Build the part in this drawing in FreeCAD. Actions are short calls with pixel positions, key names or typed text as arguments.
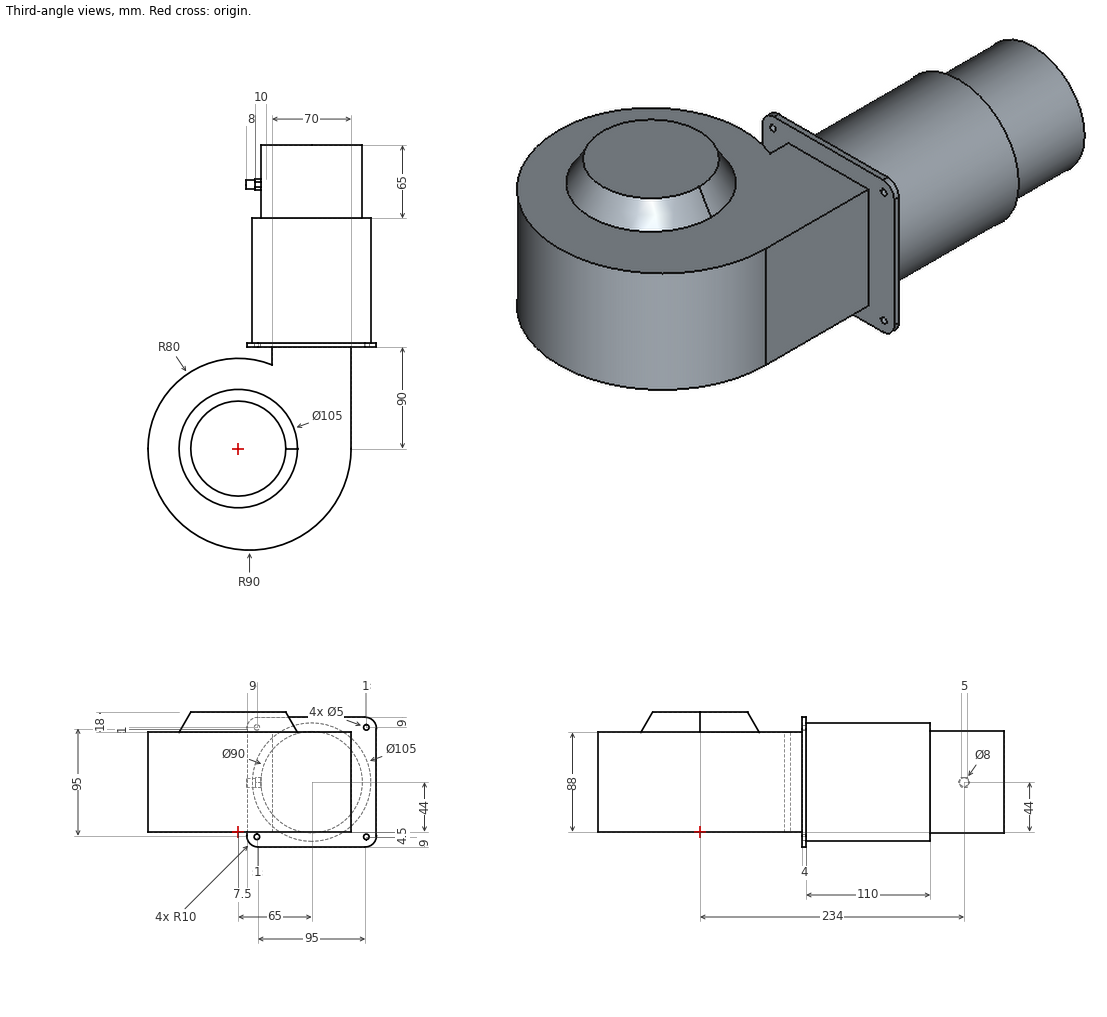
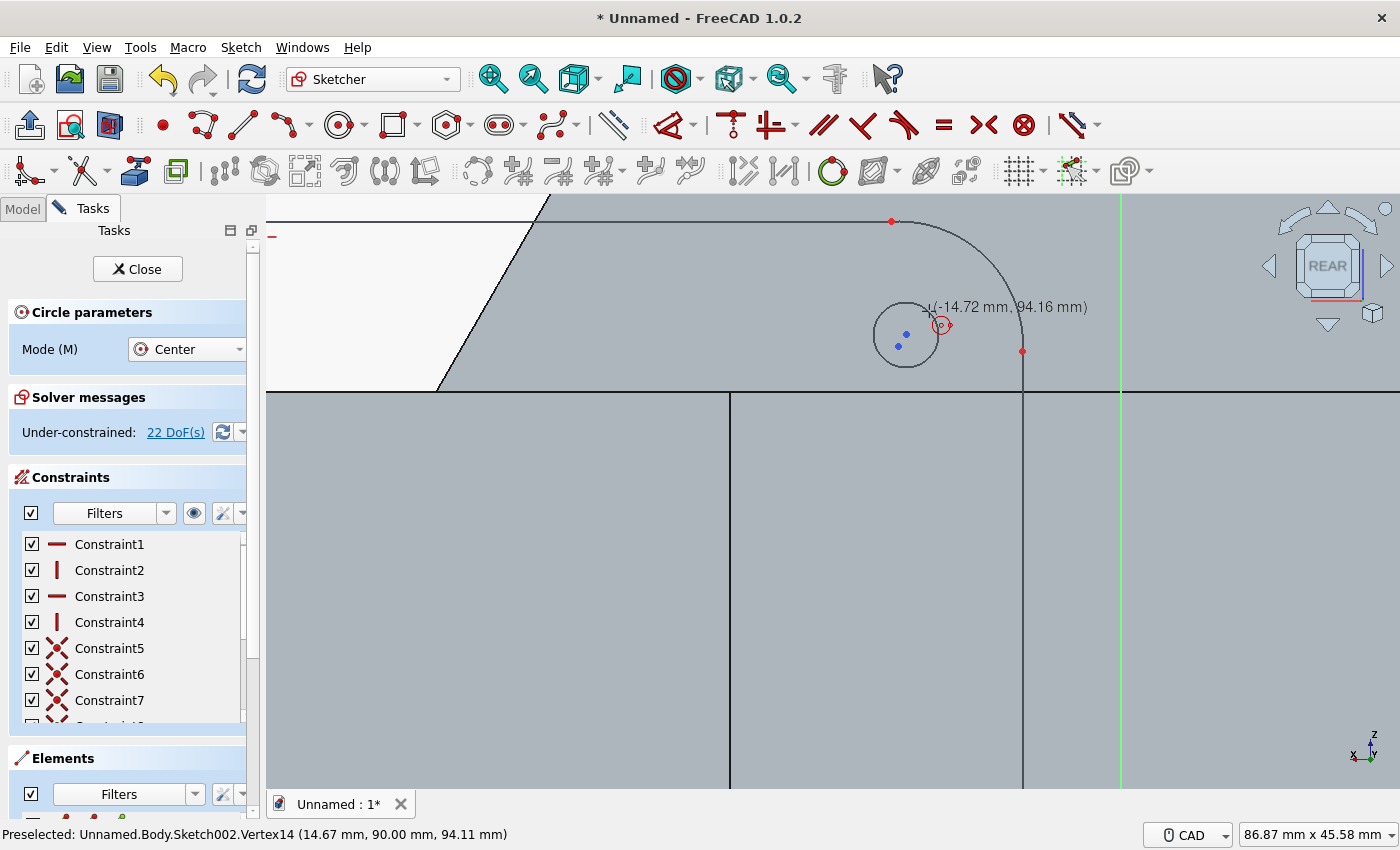
scroll(909, 336, down, 7)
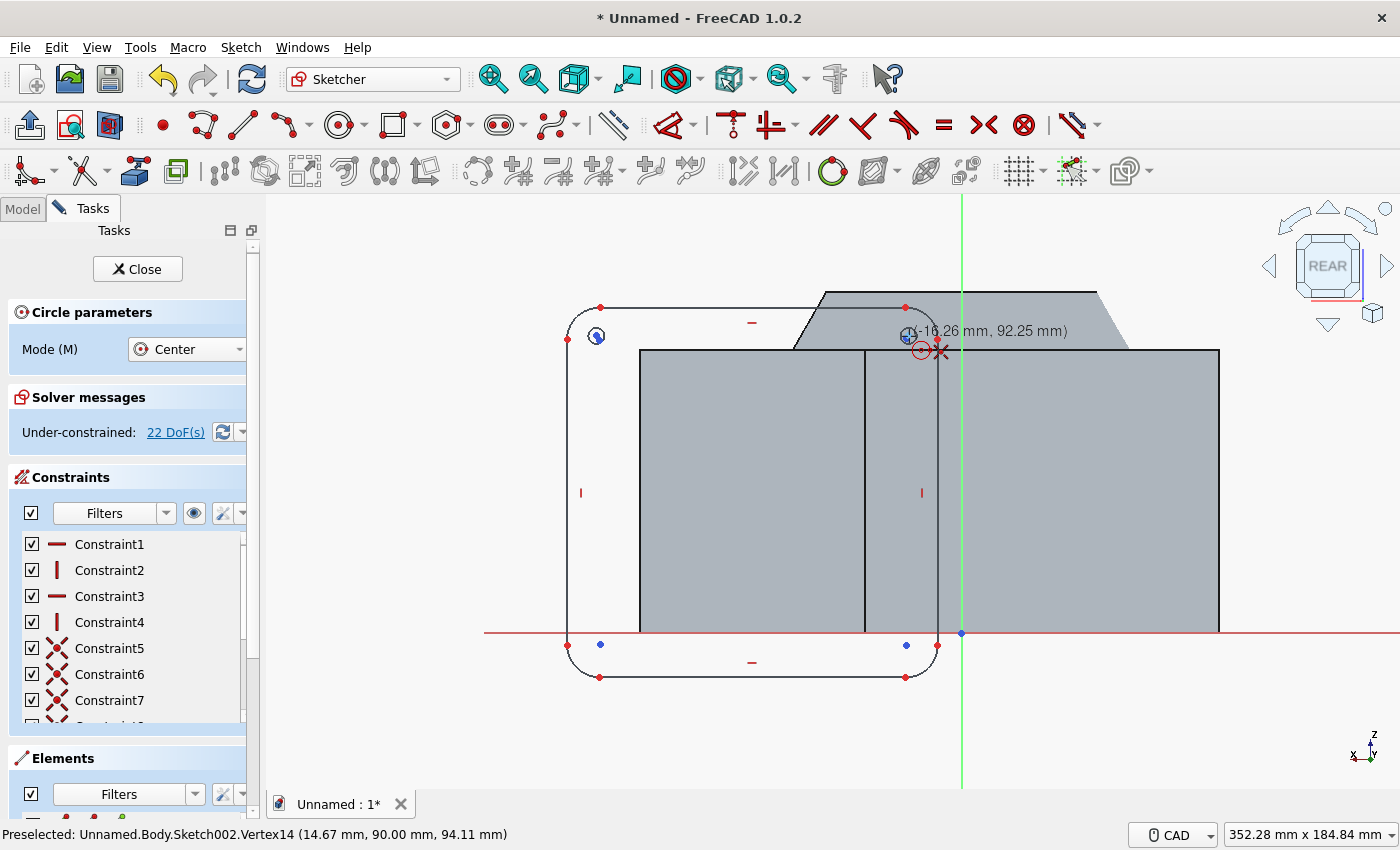
scroll(596, 648, up, 7)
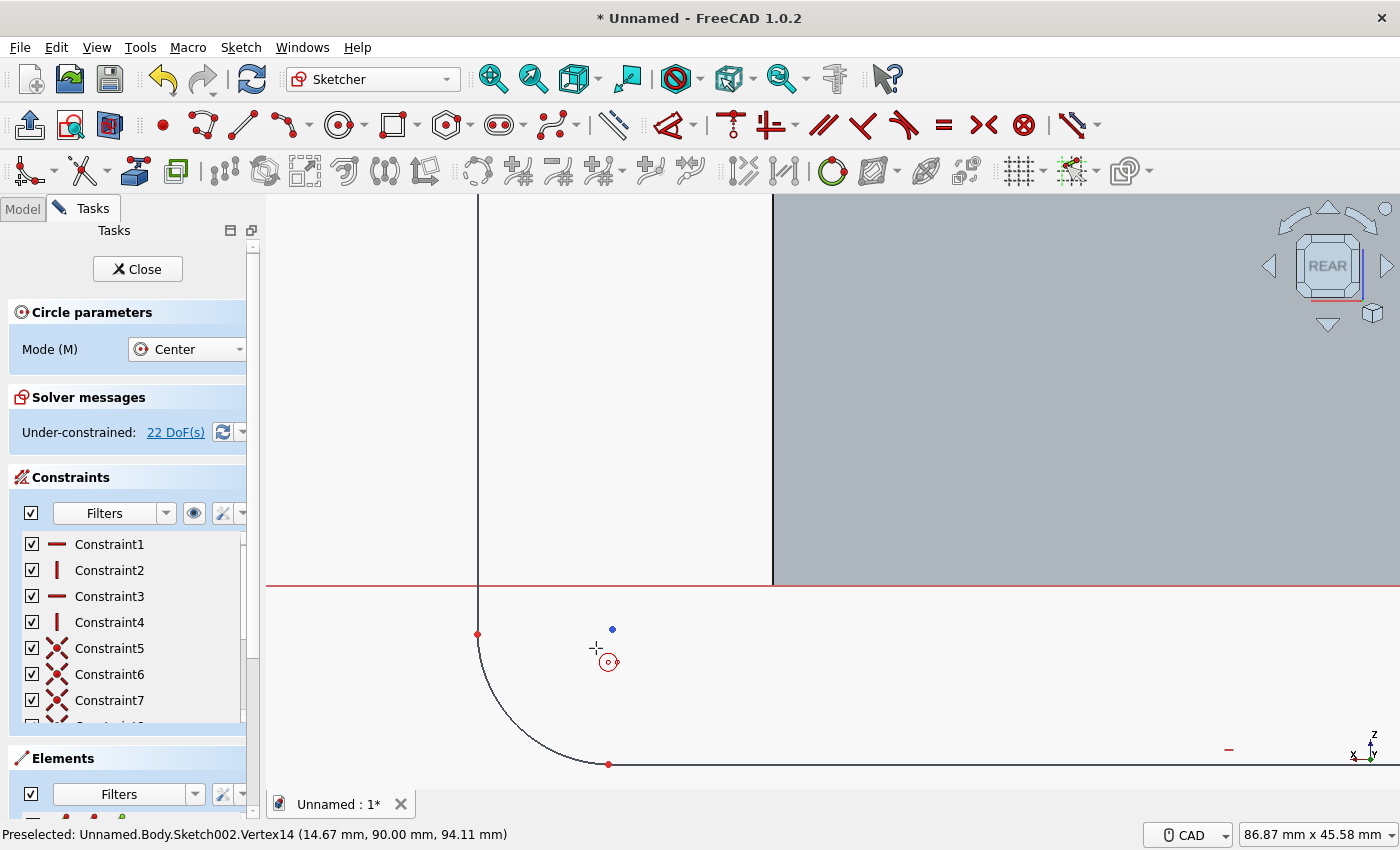
click(597, 645)
click(620, 622)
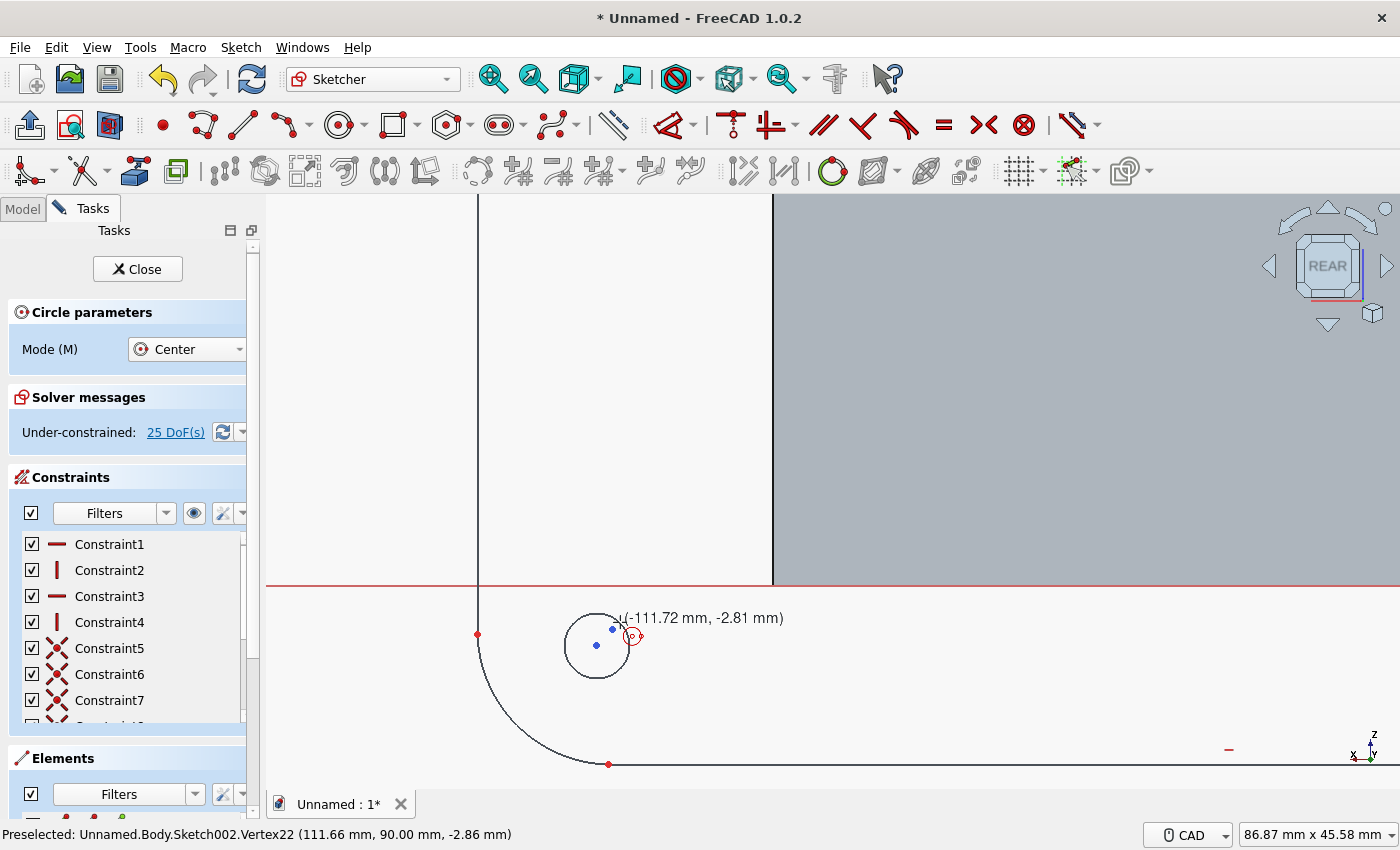
scroll(596, 648, down, 7)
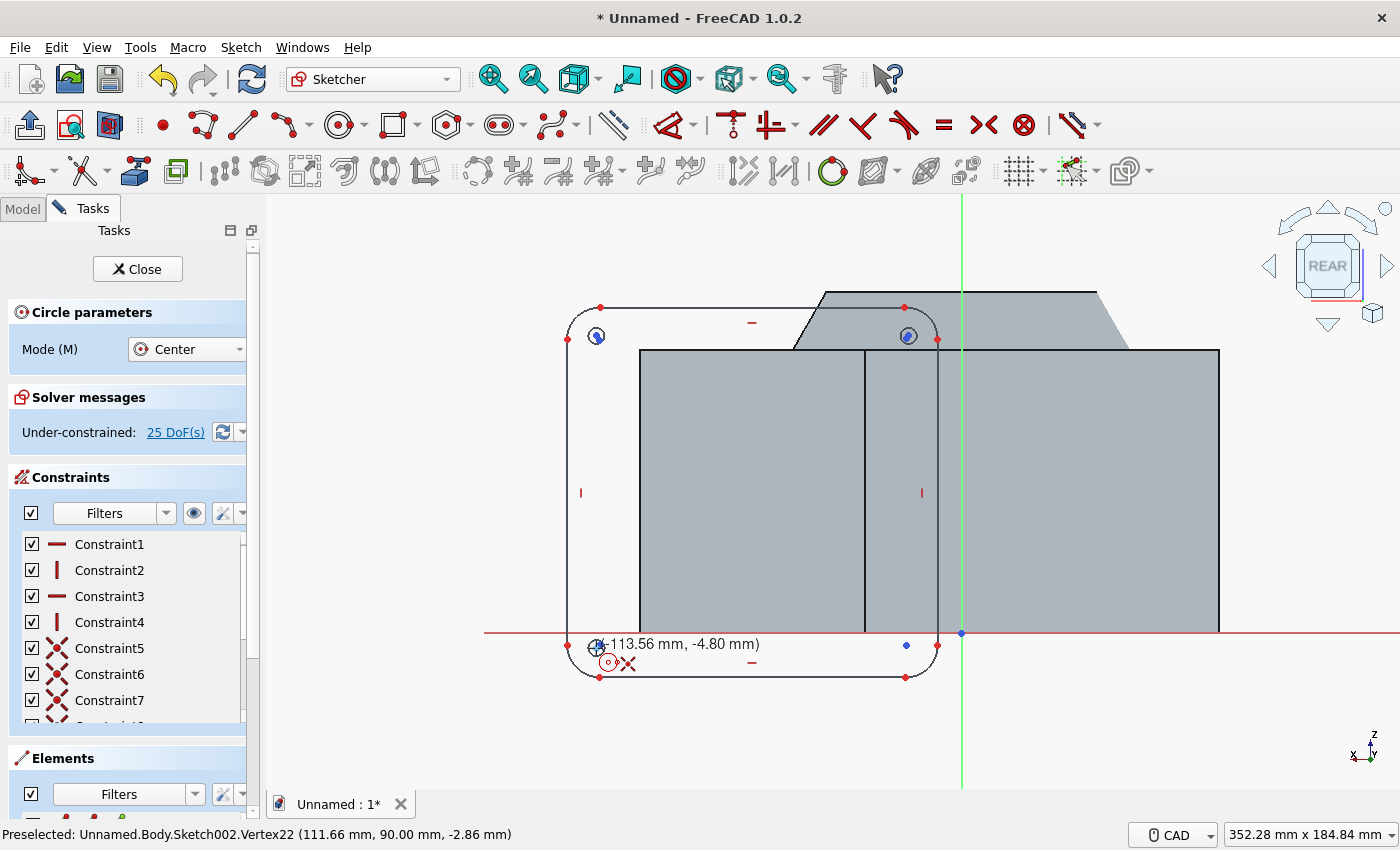
scroll(909, 648, up, 7)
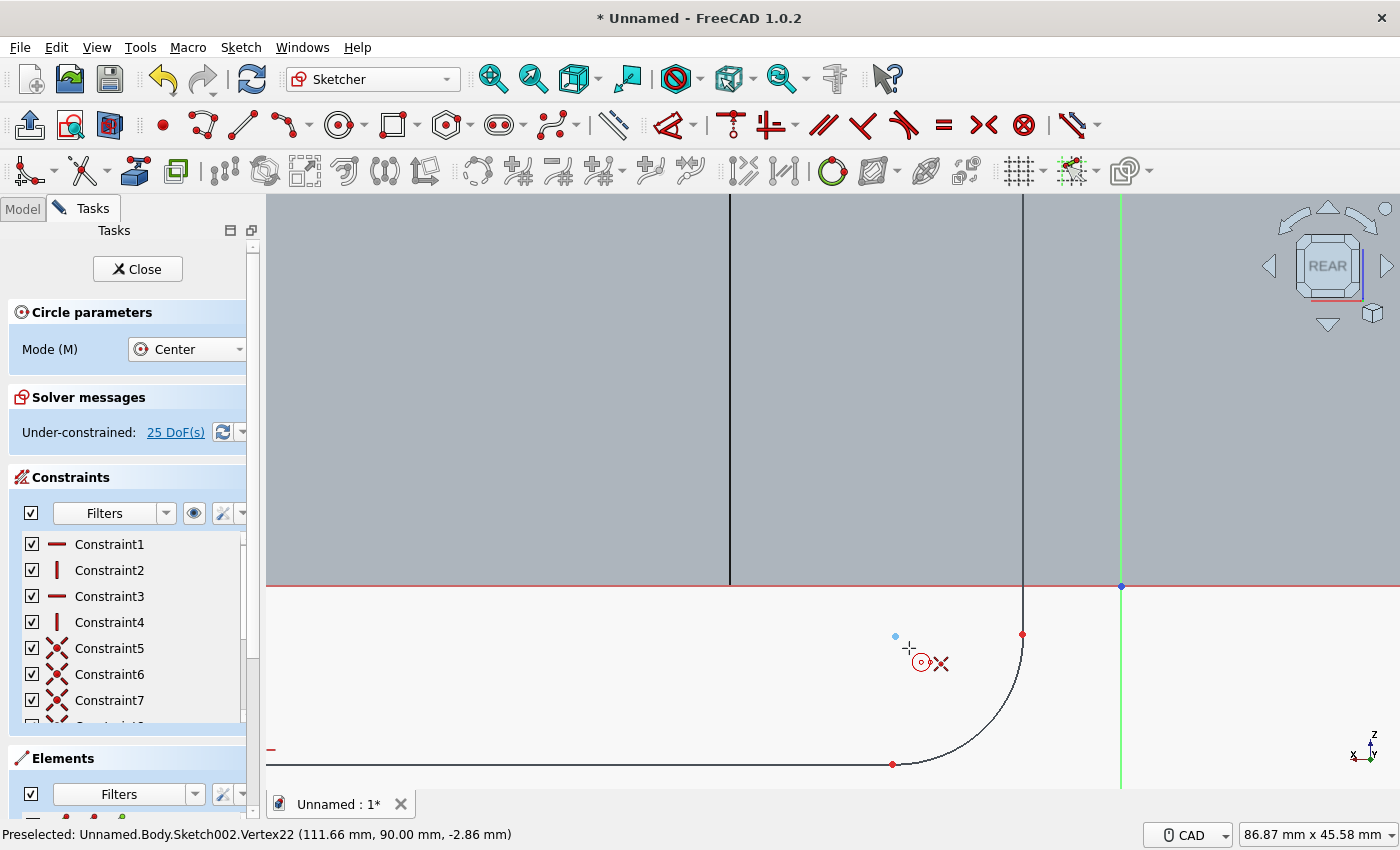
click(906, 645)
click(929, 622)
key(Escape)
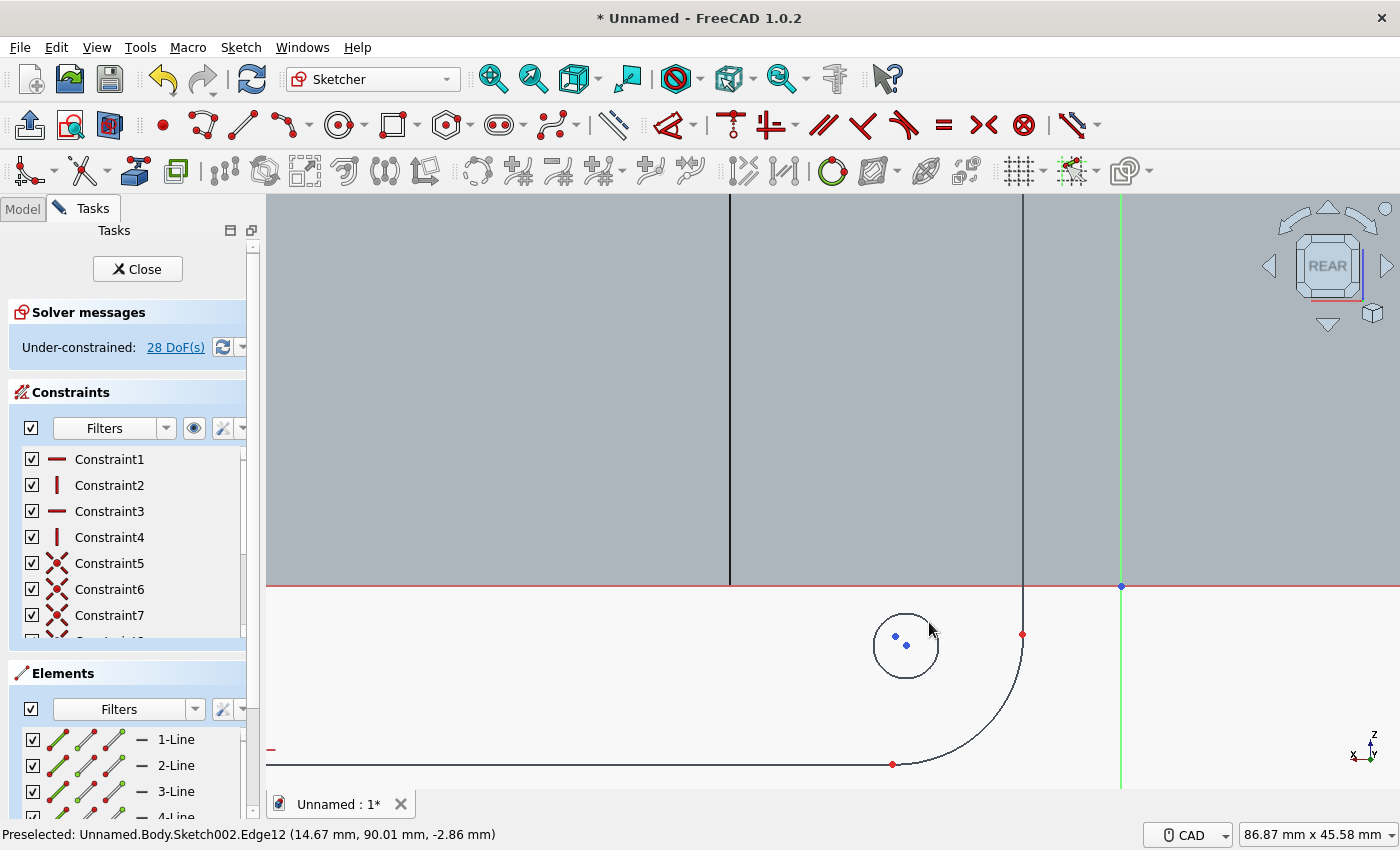
scroll(909, 648, down, 7)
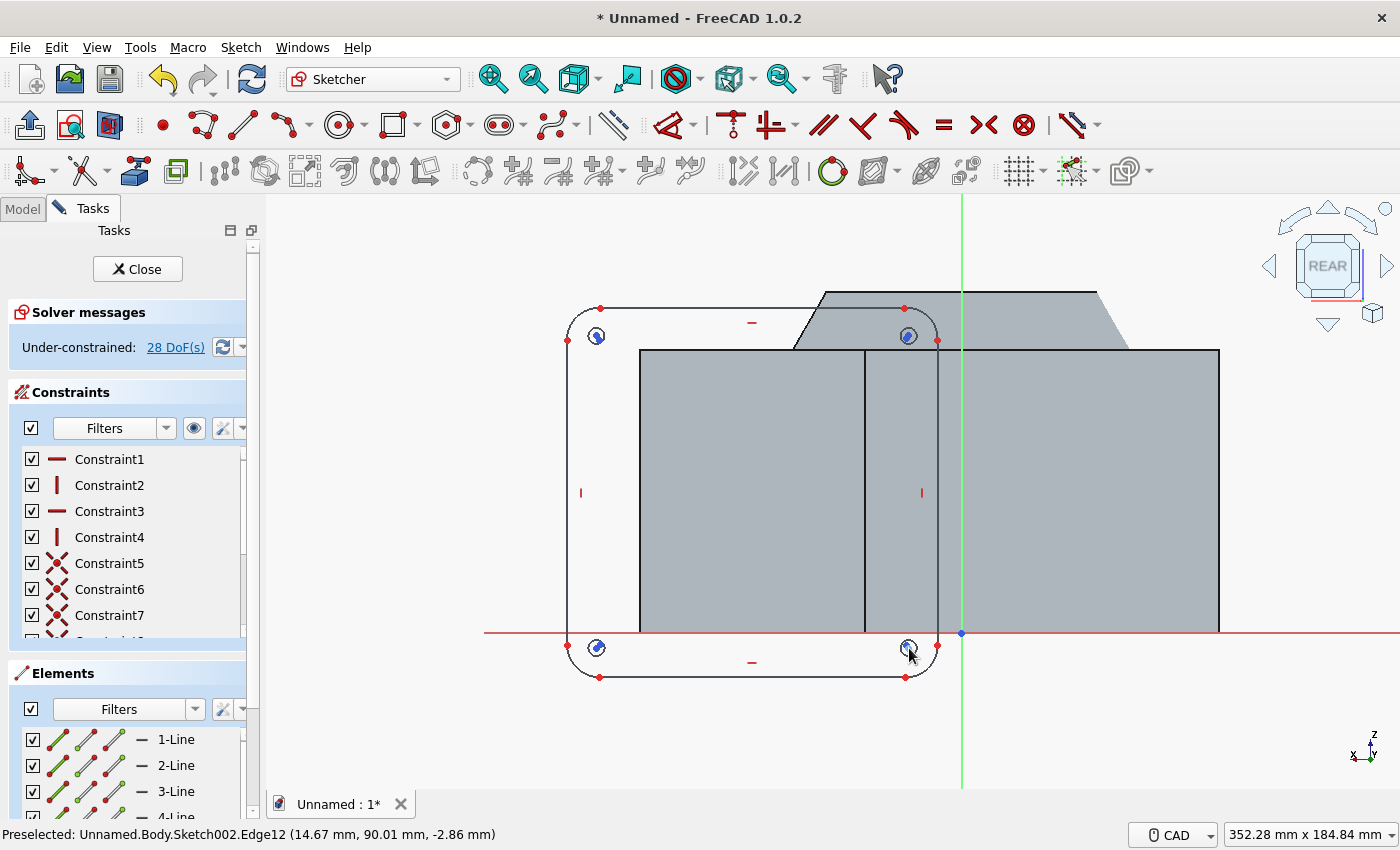
click(691, 677)